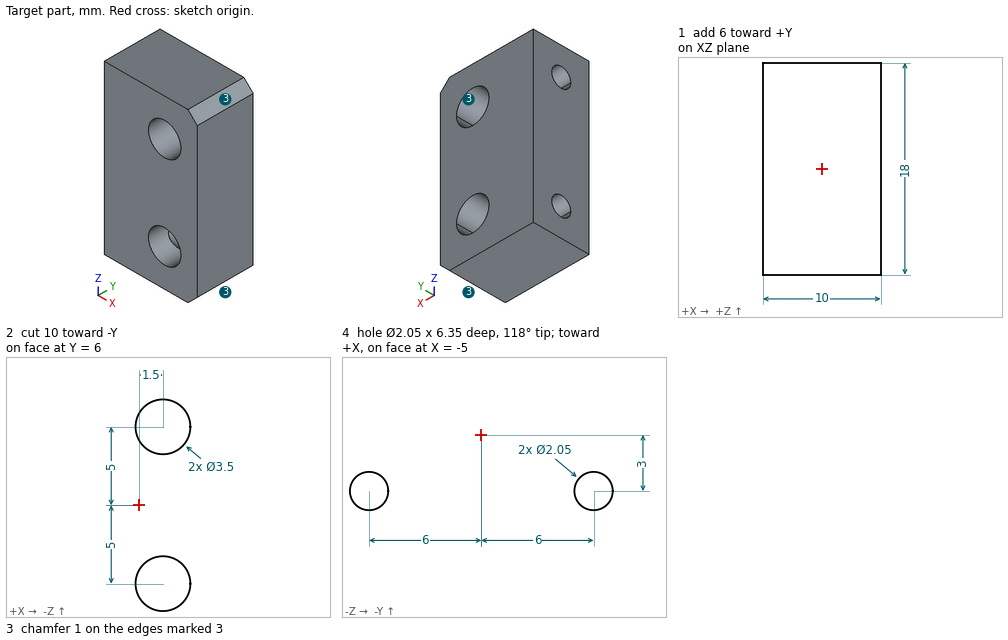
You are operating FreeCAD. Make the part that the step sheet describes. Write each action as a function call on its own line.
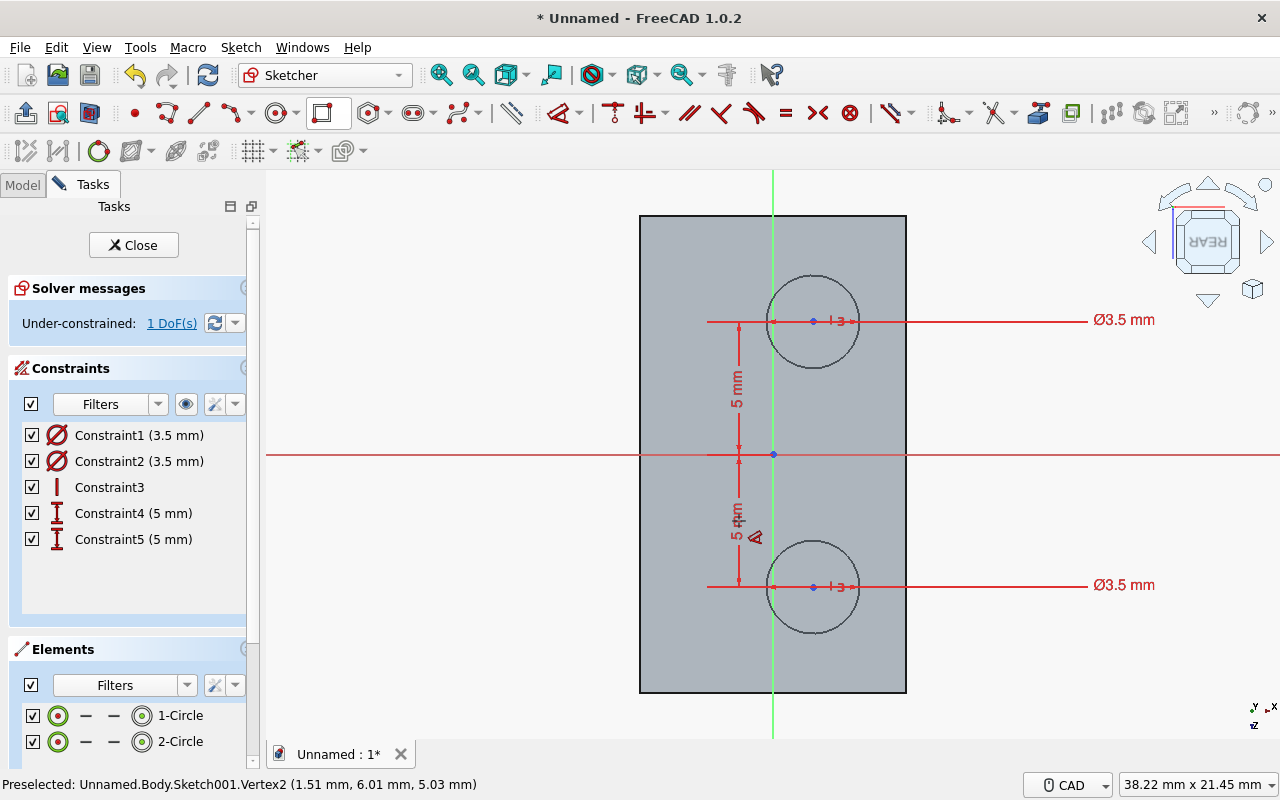
click(813, 322)
click(793, 489)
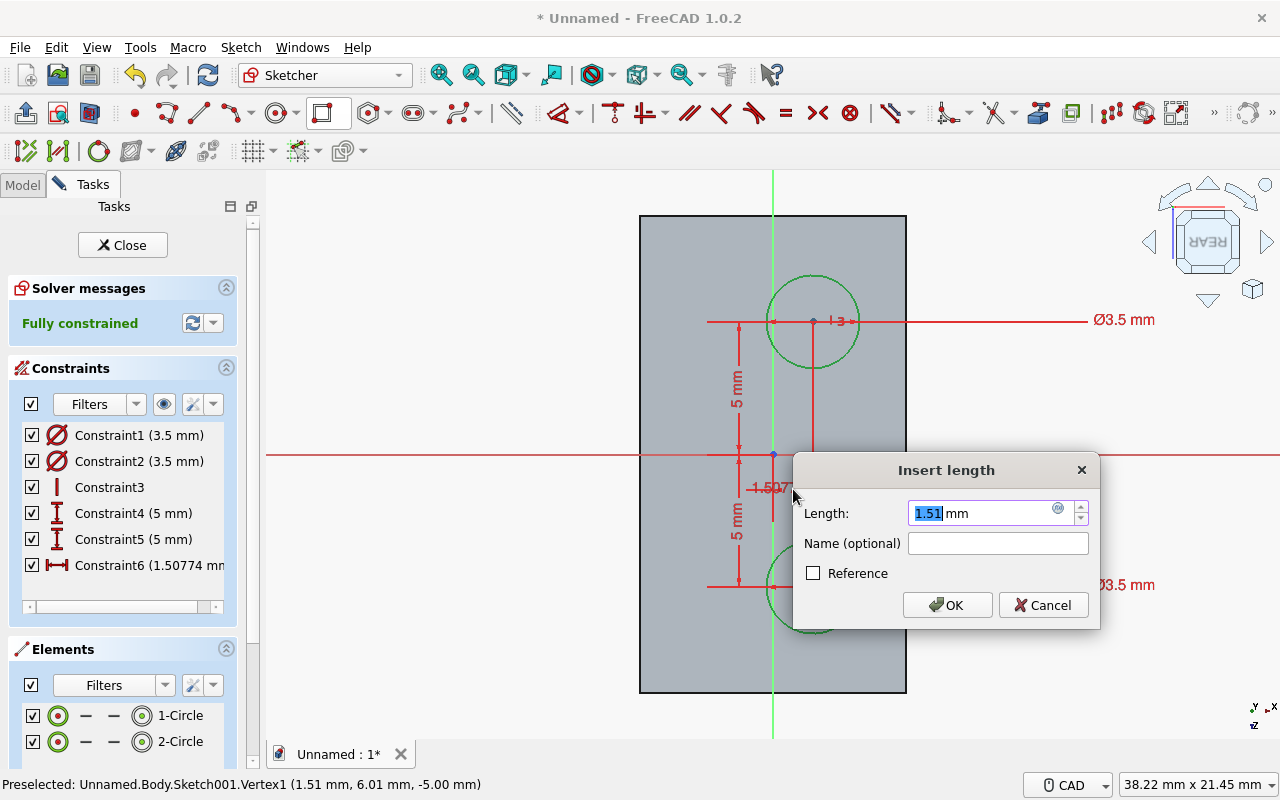
text(1.5)
key(Return)
key(Escape)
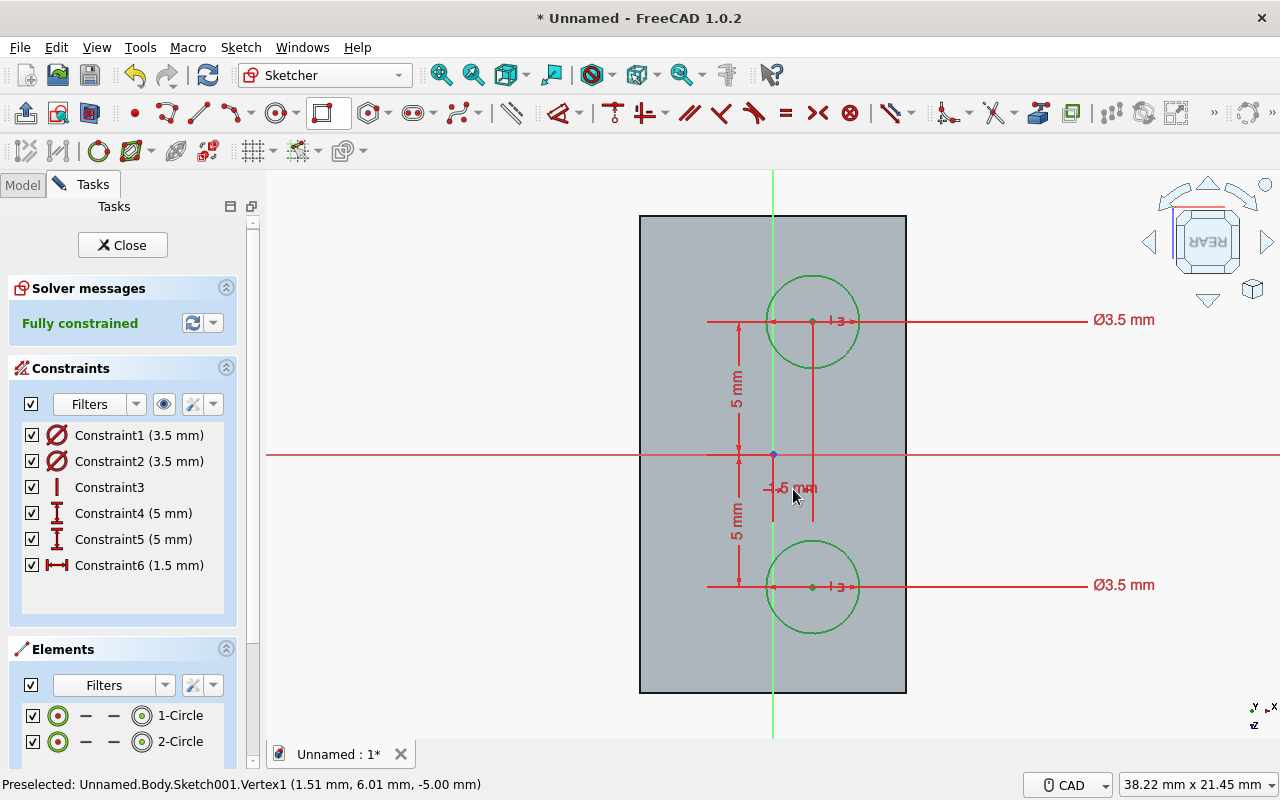
click(123, 245)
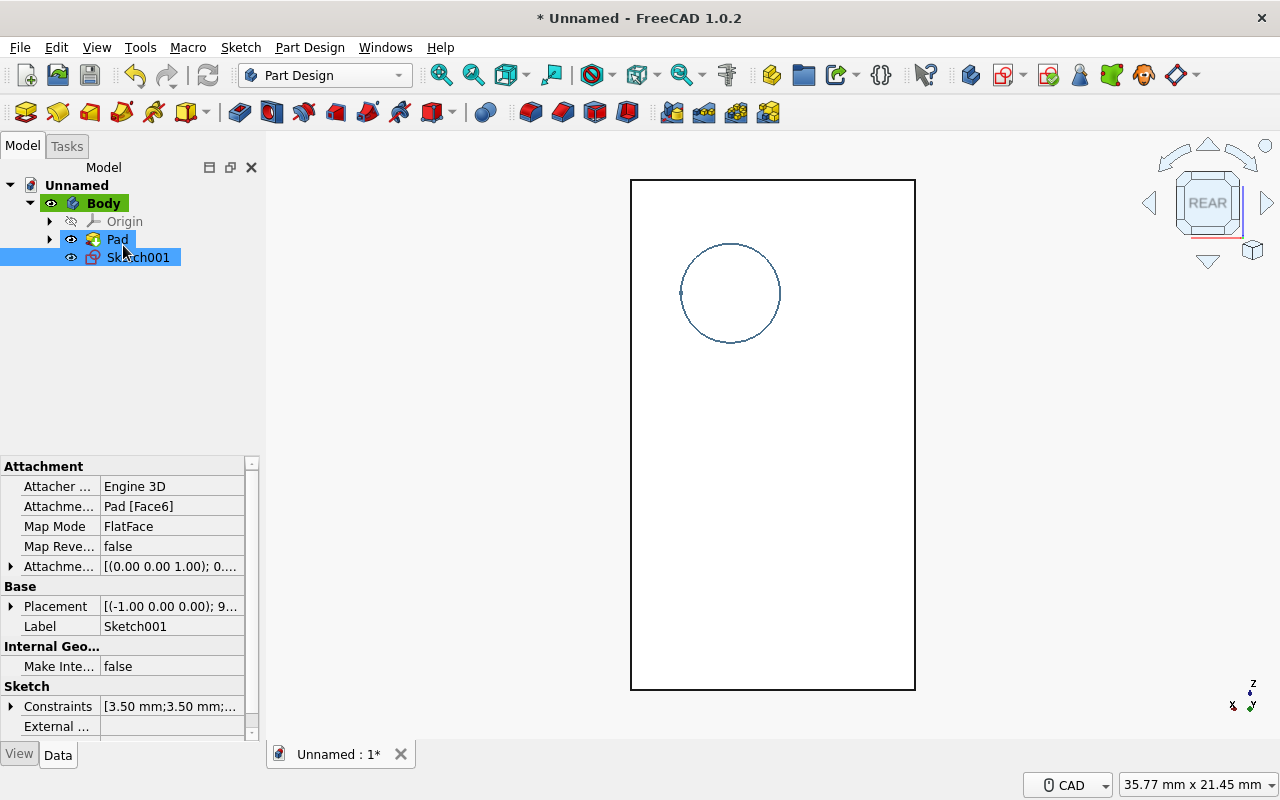
click(240, 112)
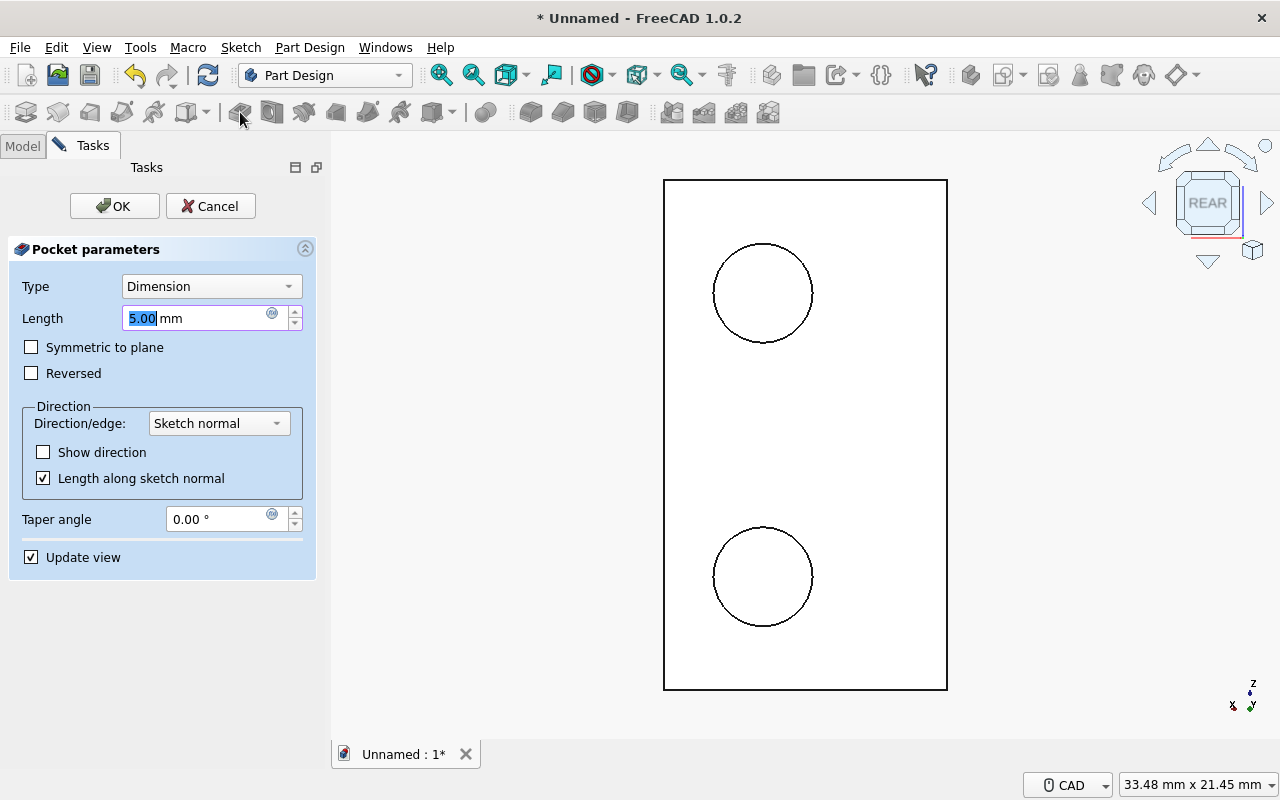
text(10)
key(Tab)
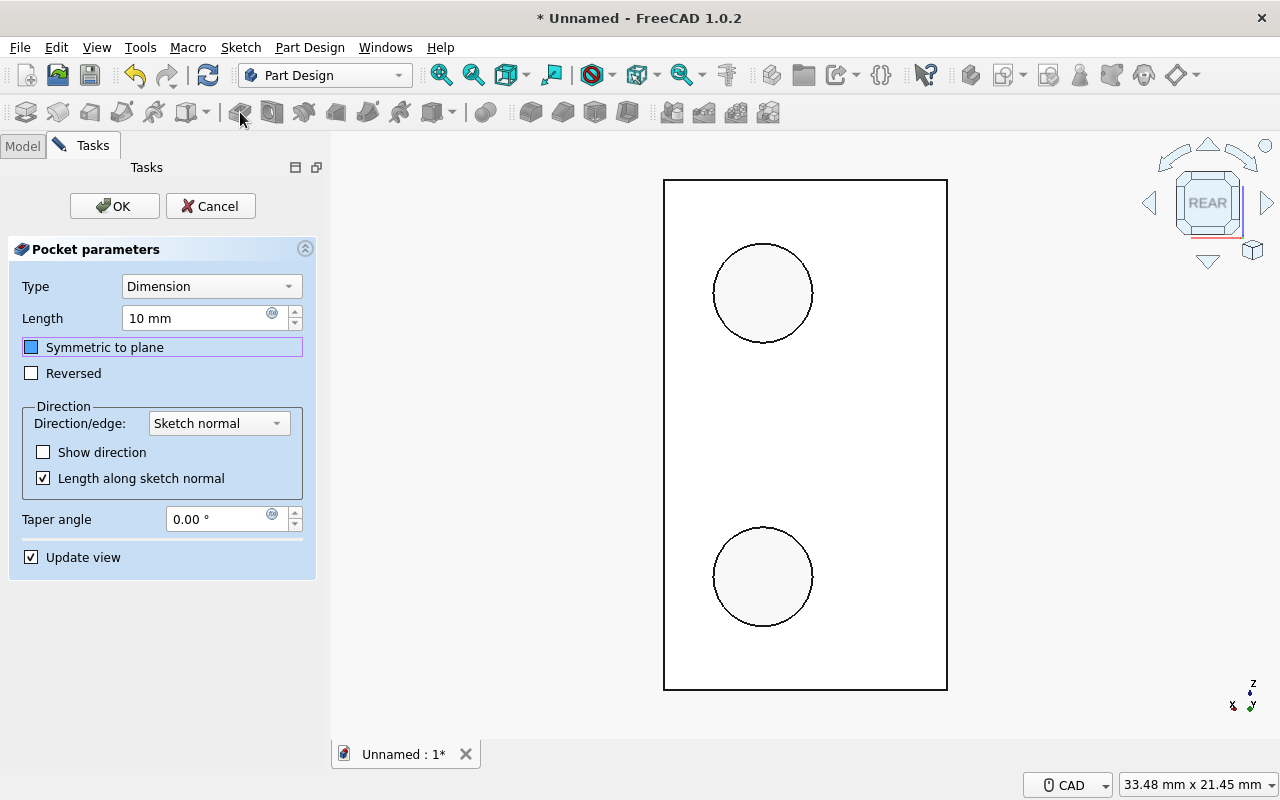
click(115, 206)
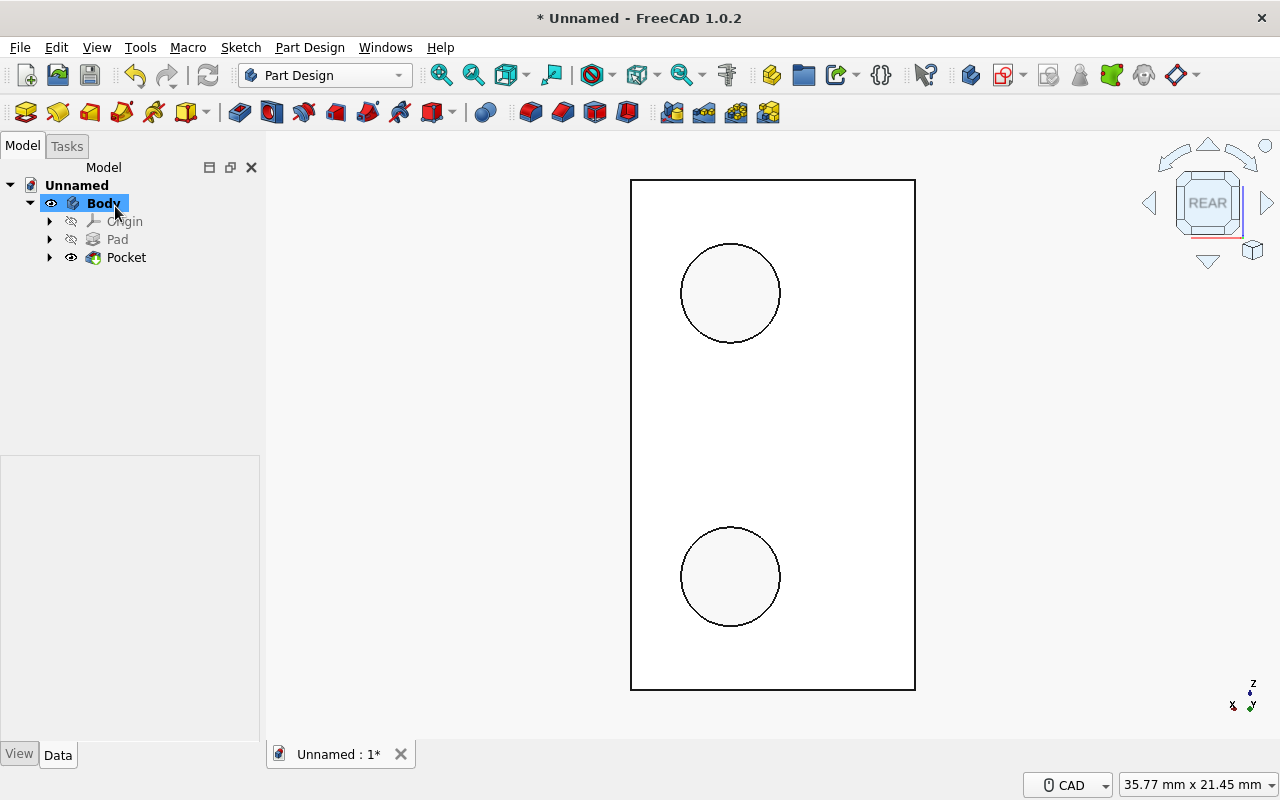
key(0)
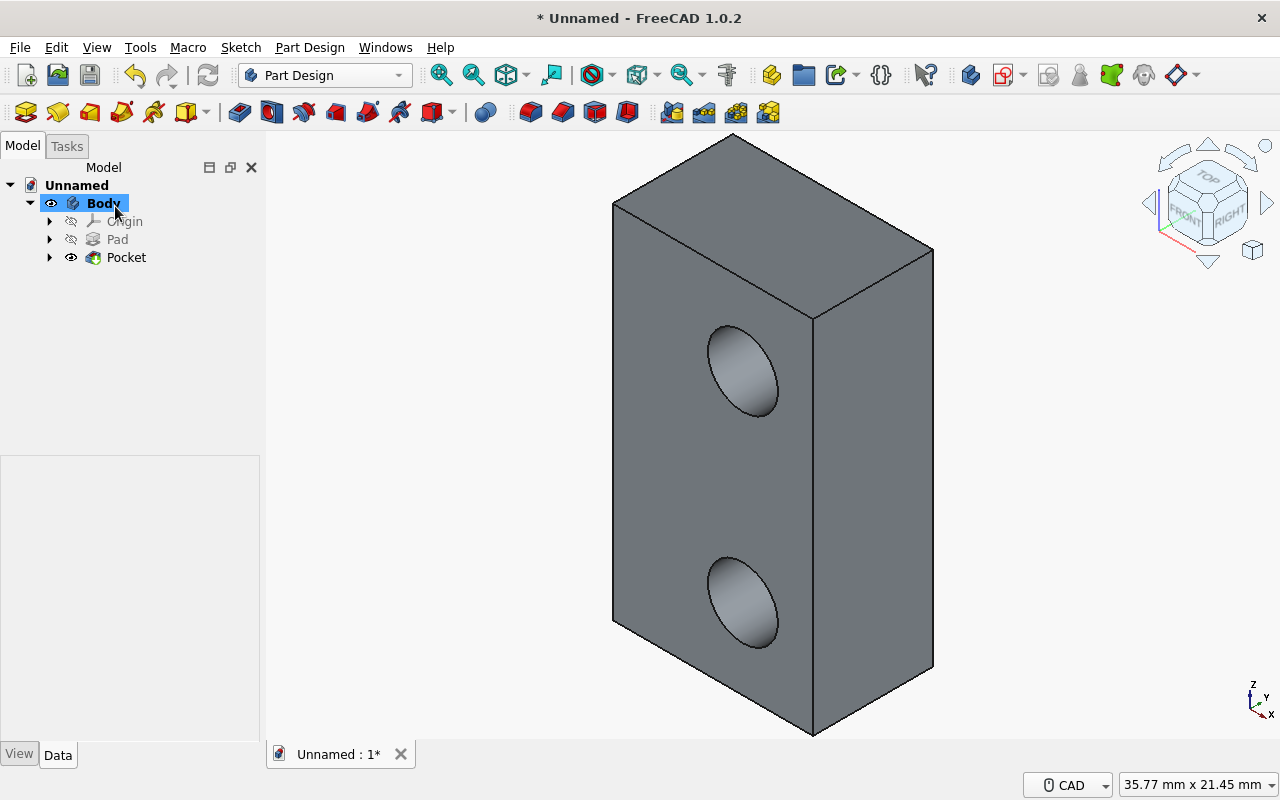
click(873, 284)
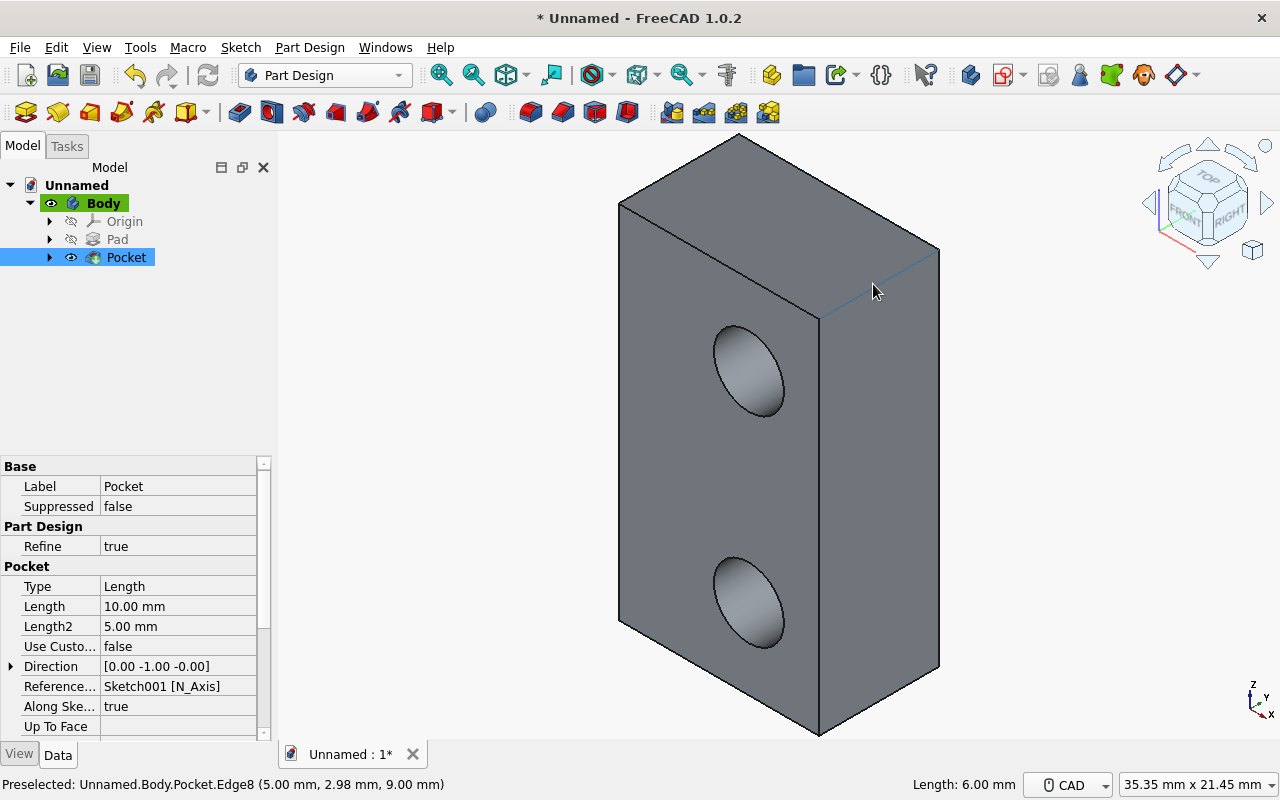
key(2)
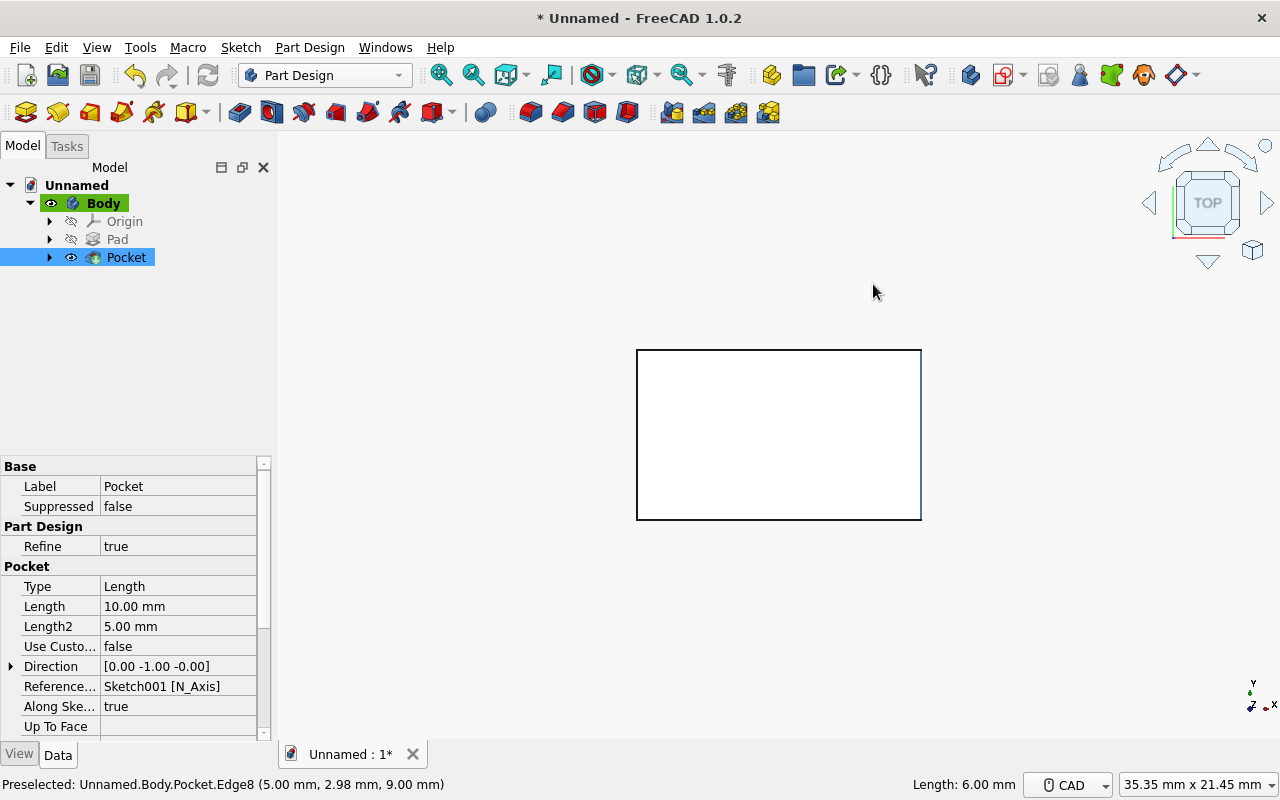
key(v)
key(f)